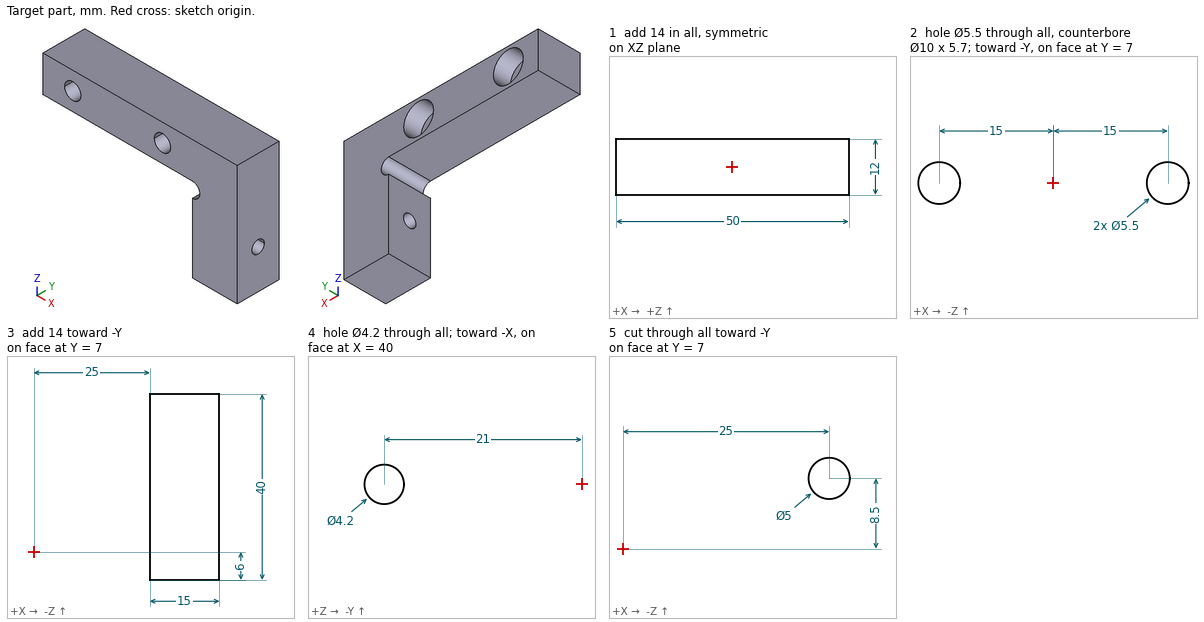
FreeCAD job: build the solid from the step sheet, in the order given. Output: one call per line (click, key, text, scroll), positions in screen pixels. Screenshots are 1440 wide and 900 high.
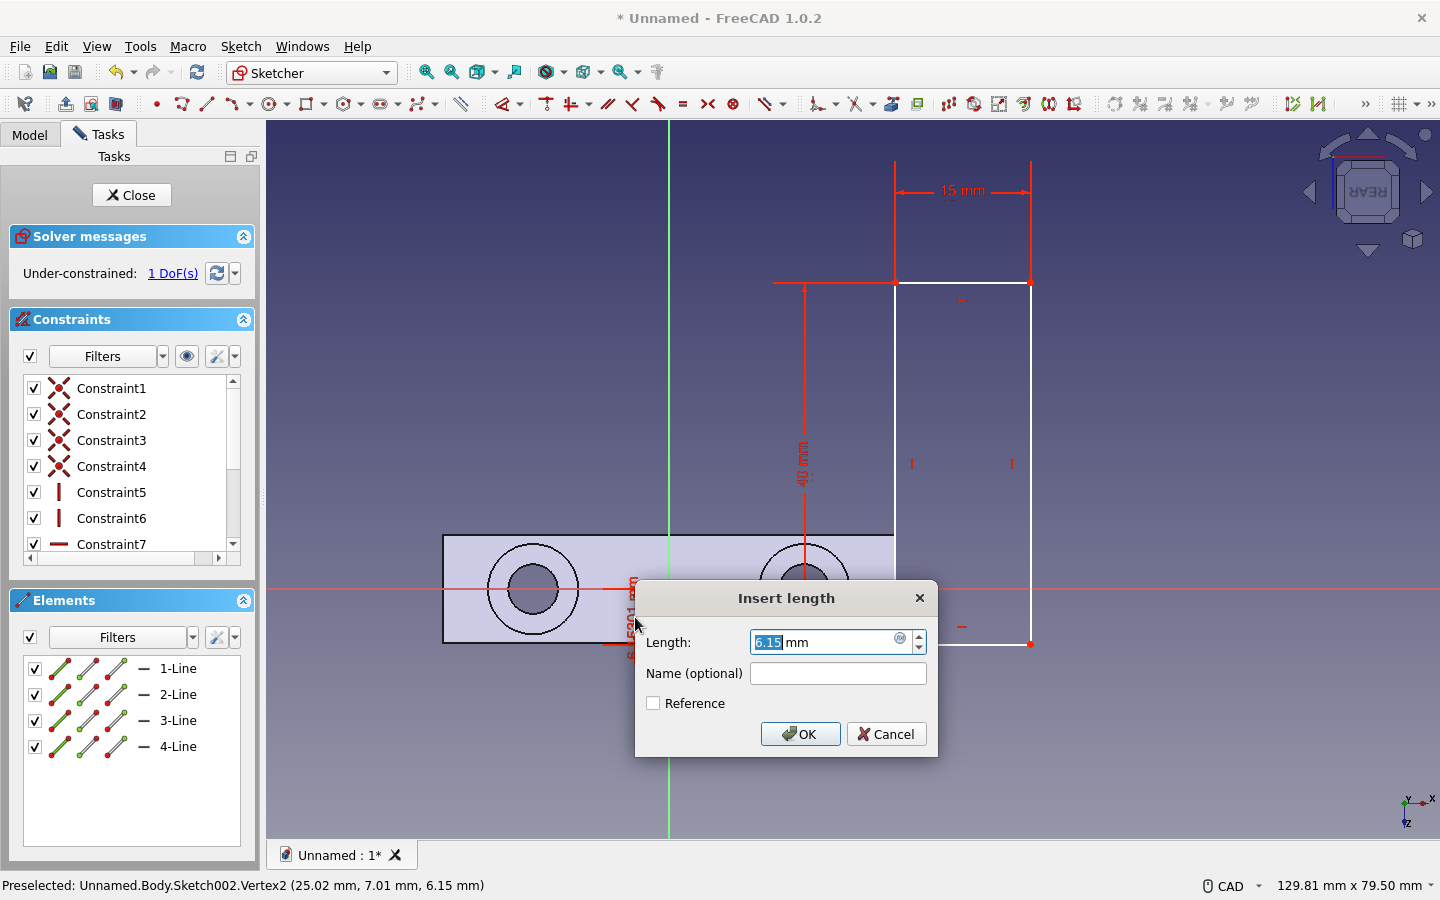
text(6)
key(Return)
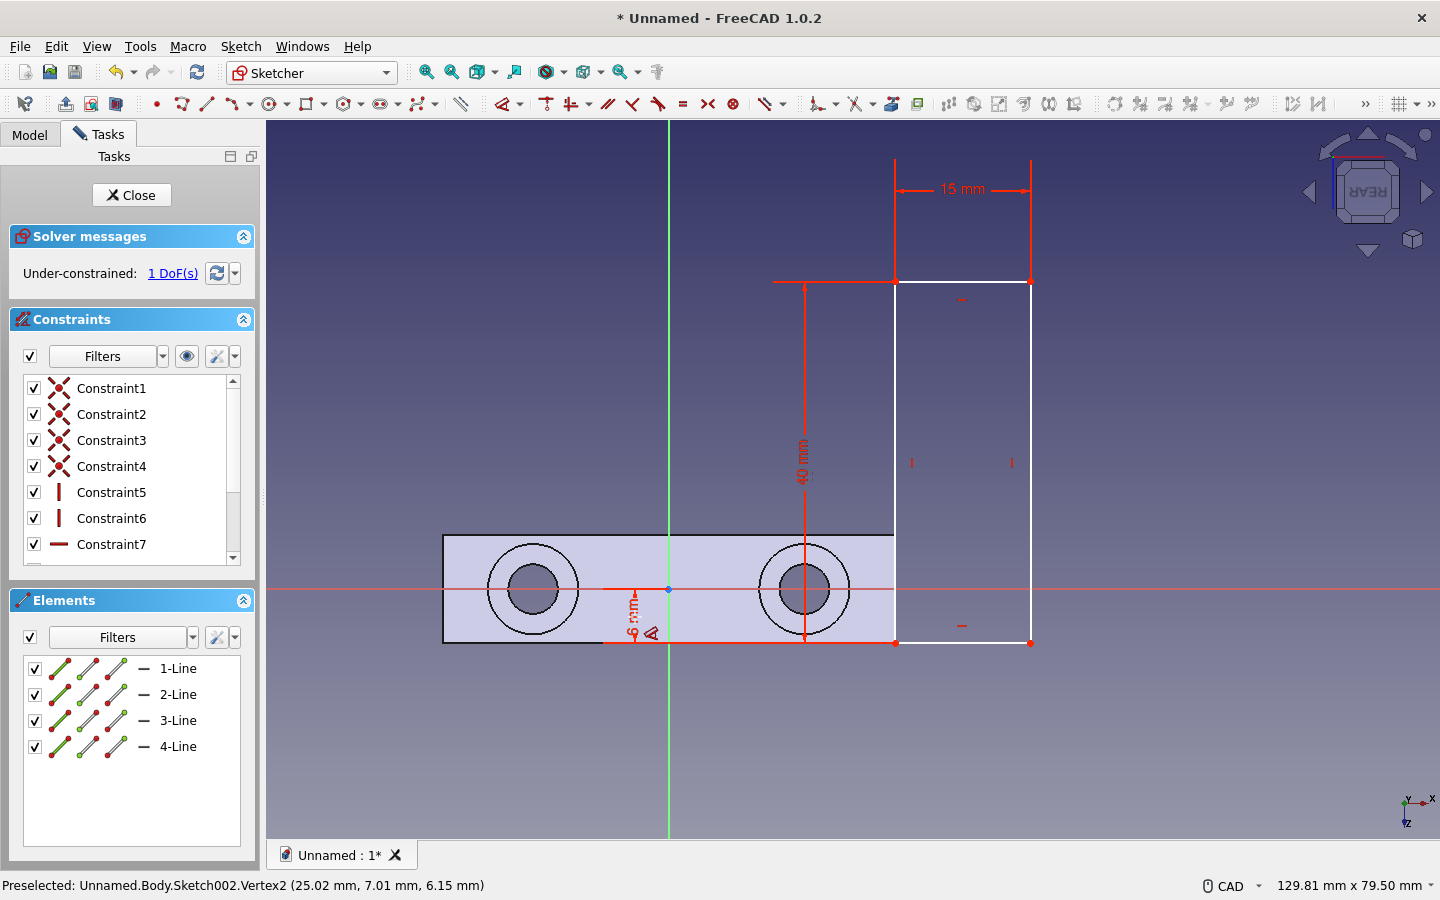
click(895, 282)
click(782, 248)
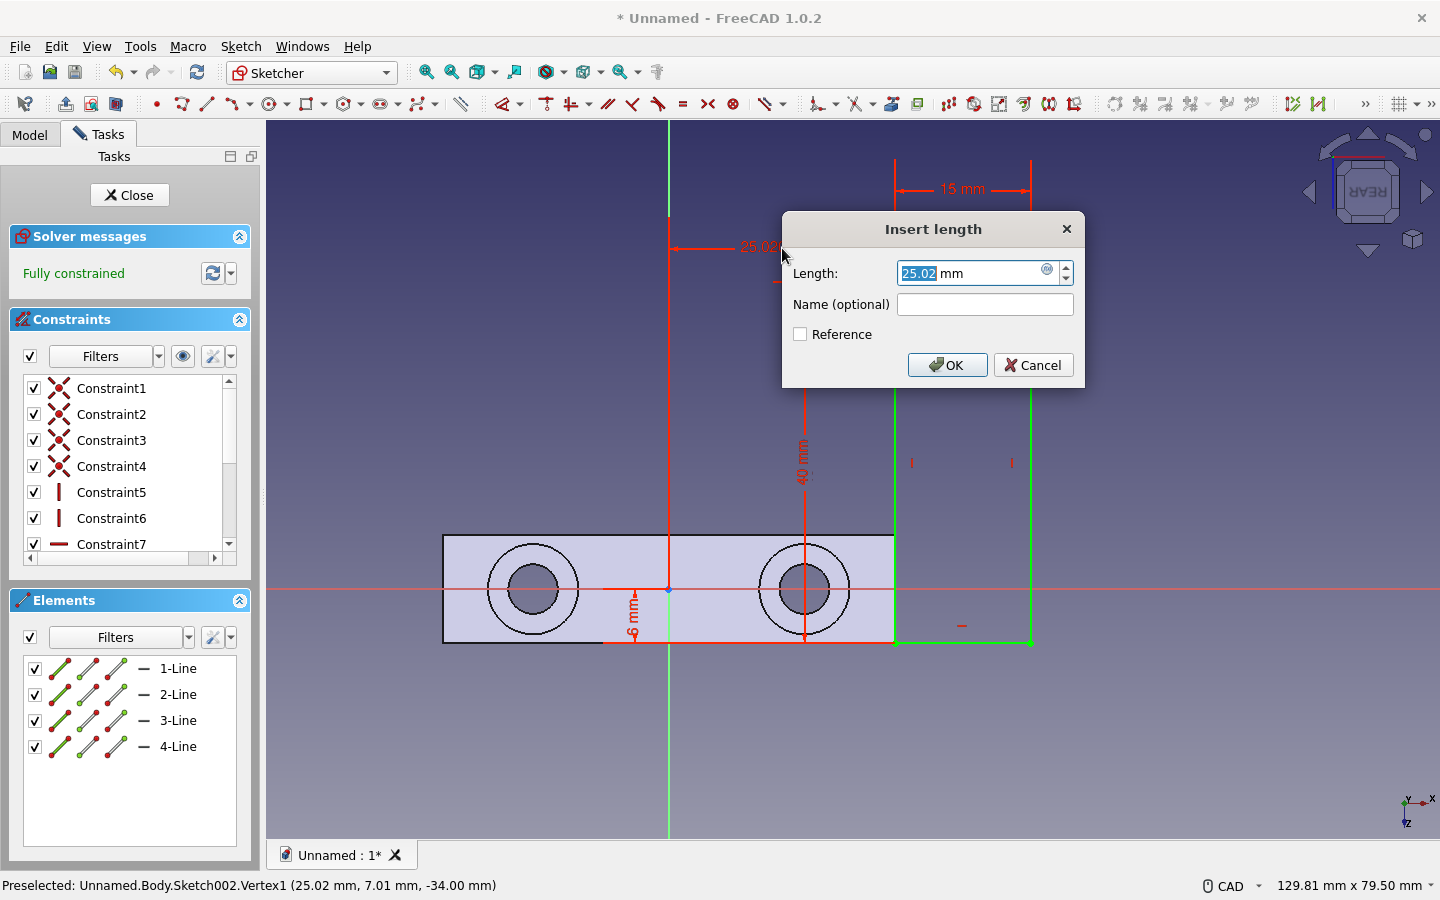
text(25)
key(Return)
key(Escape)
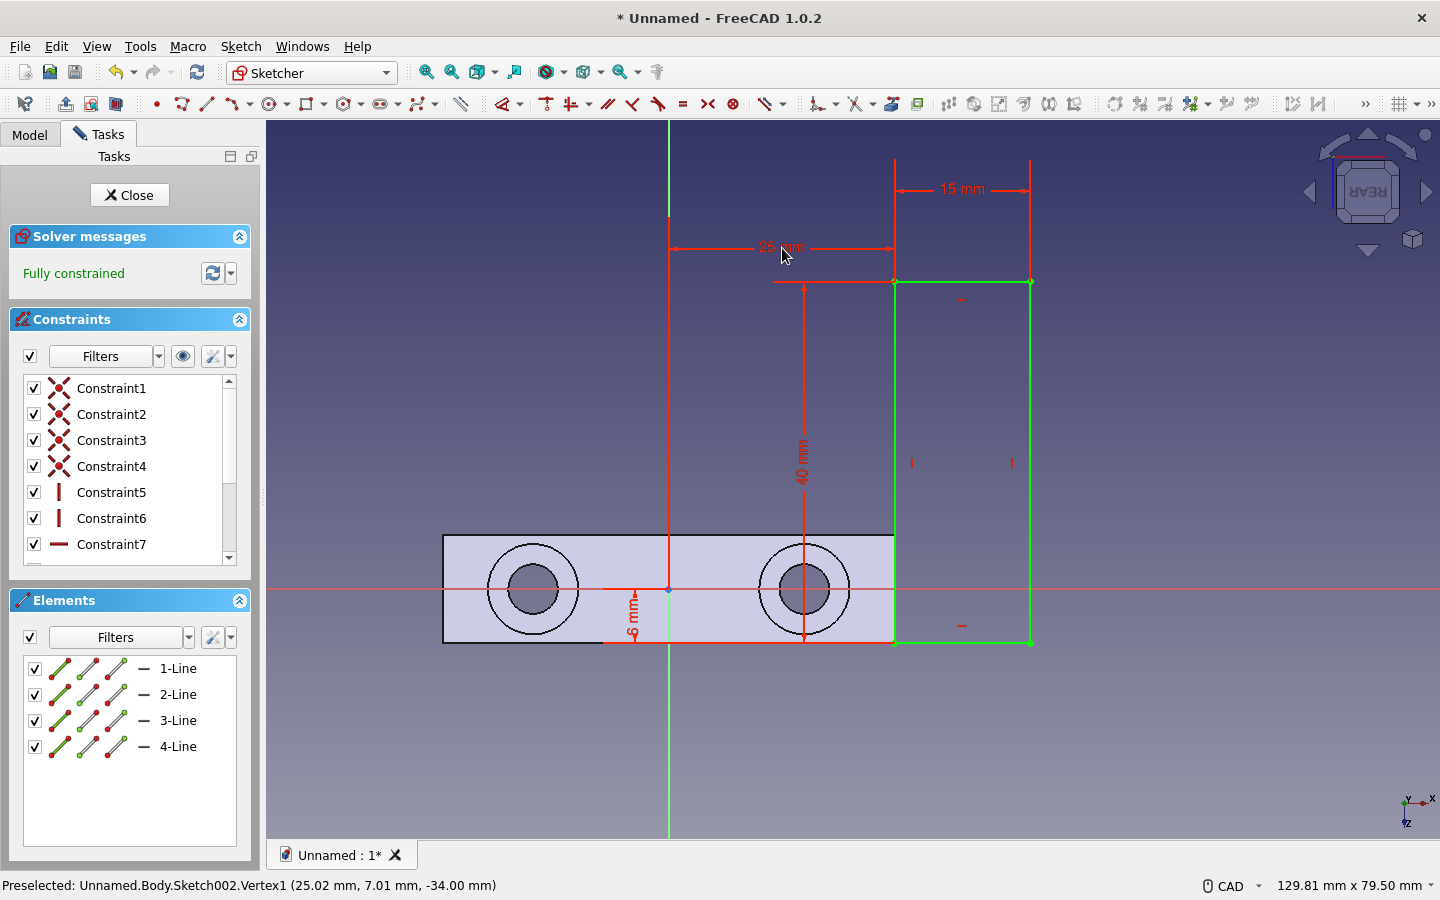
click(130, 195)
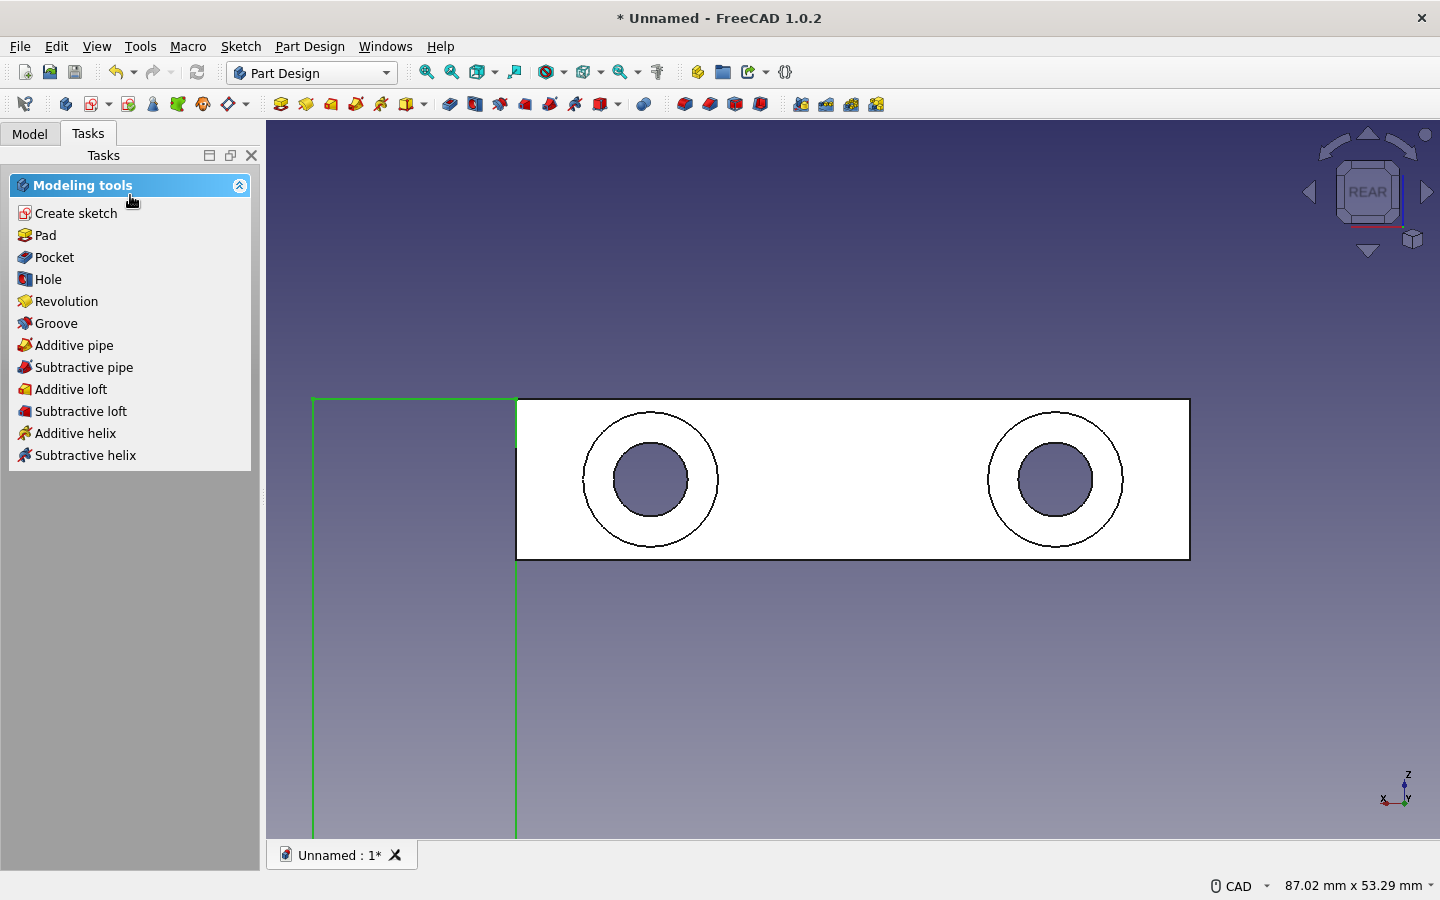
click(281, 104)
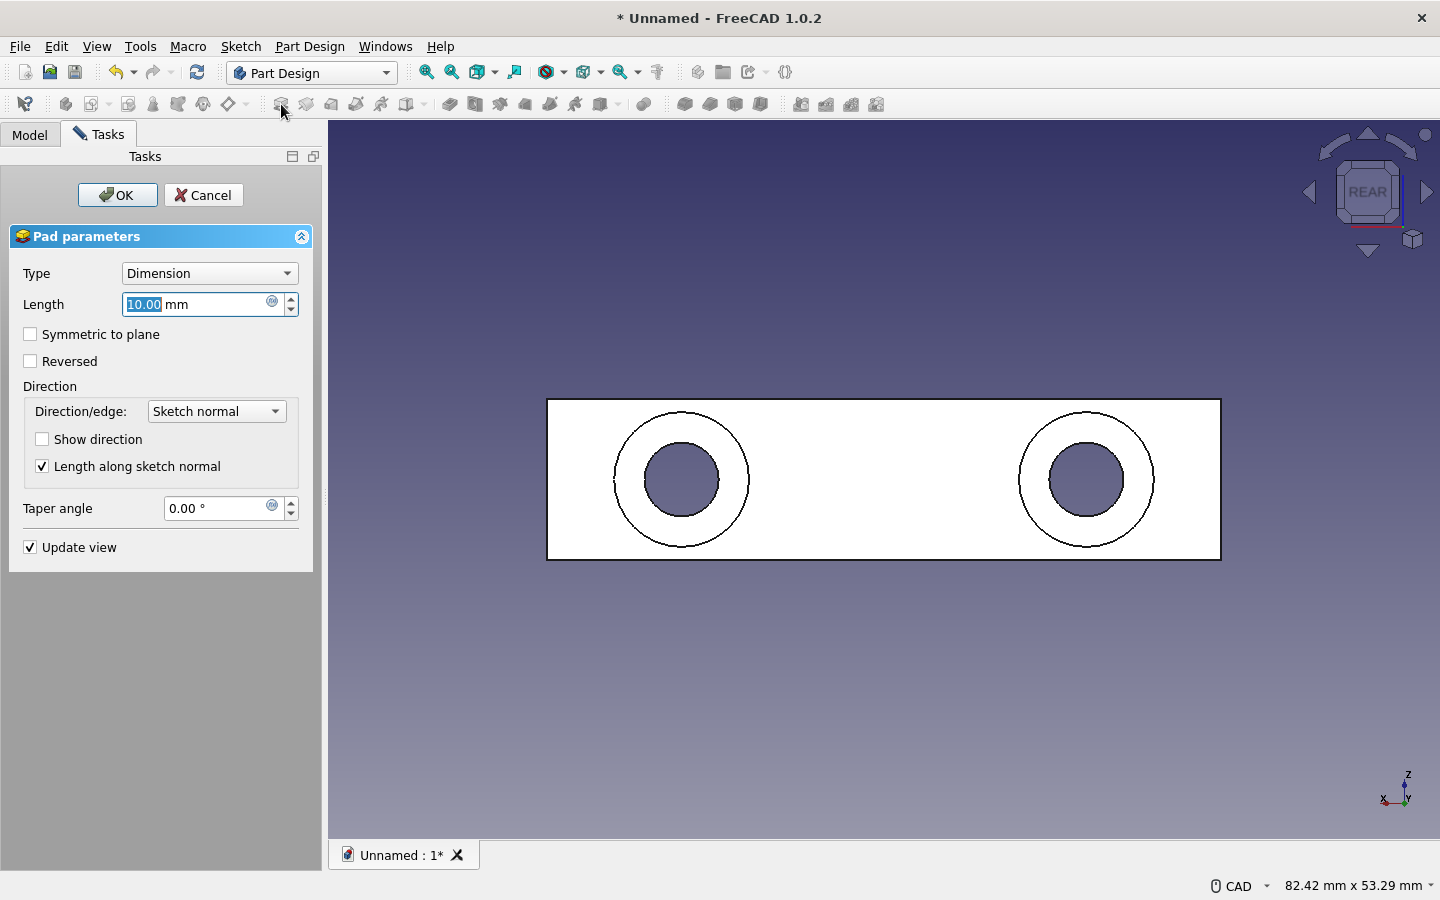
text(14)
key(Tab)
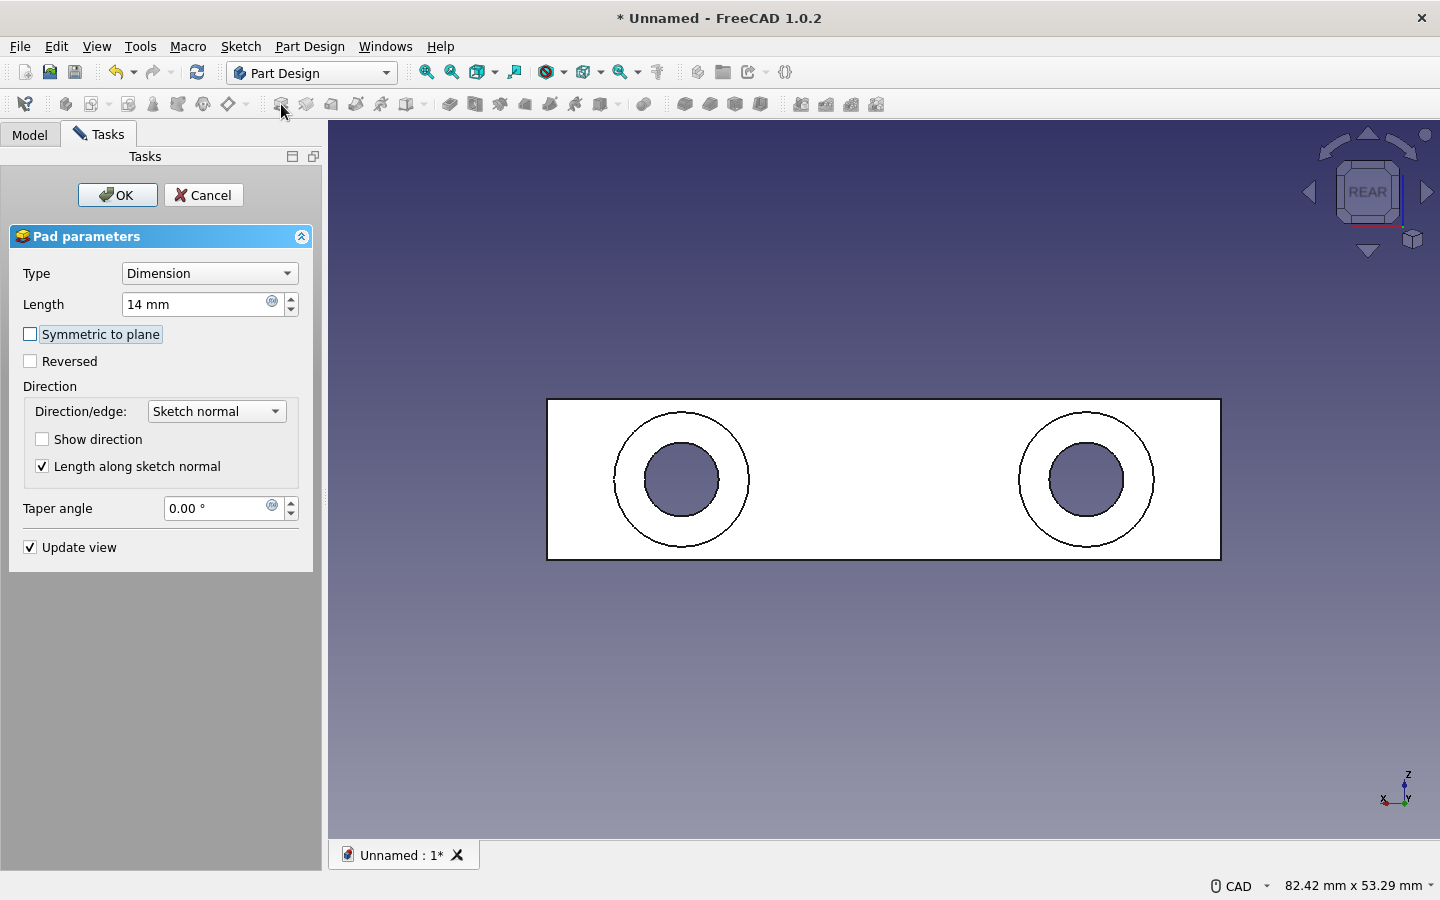
click(31, 361)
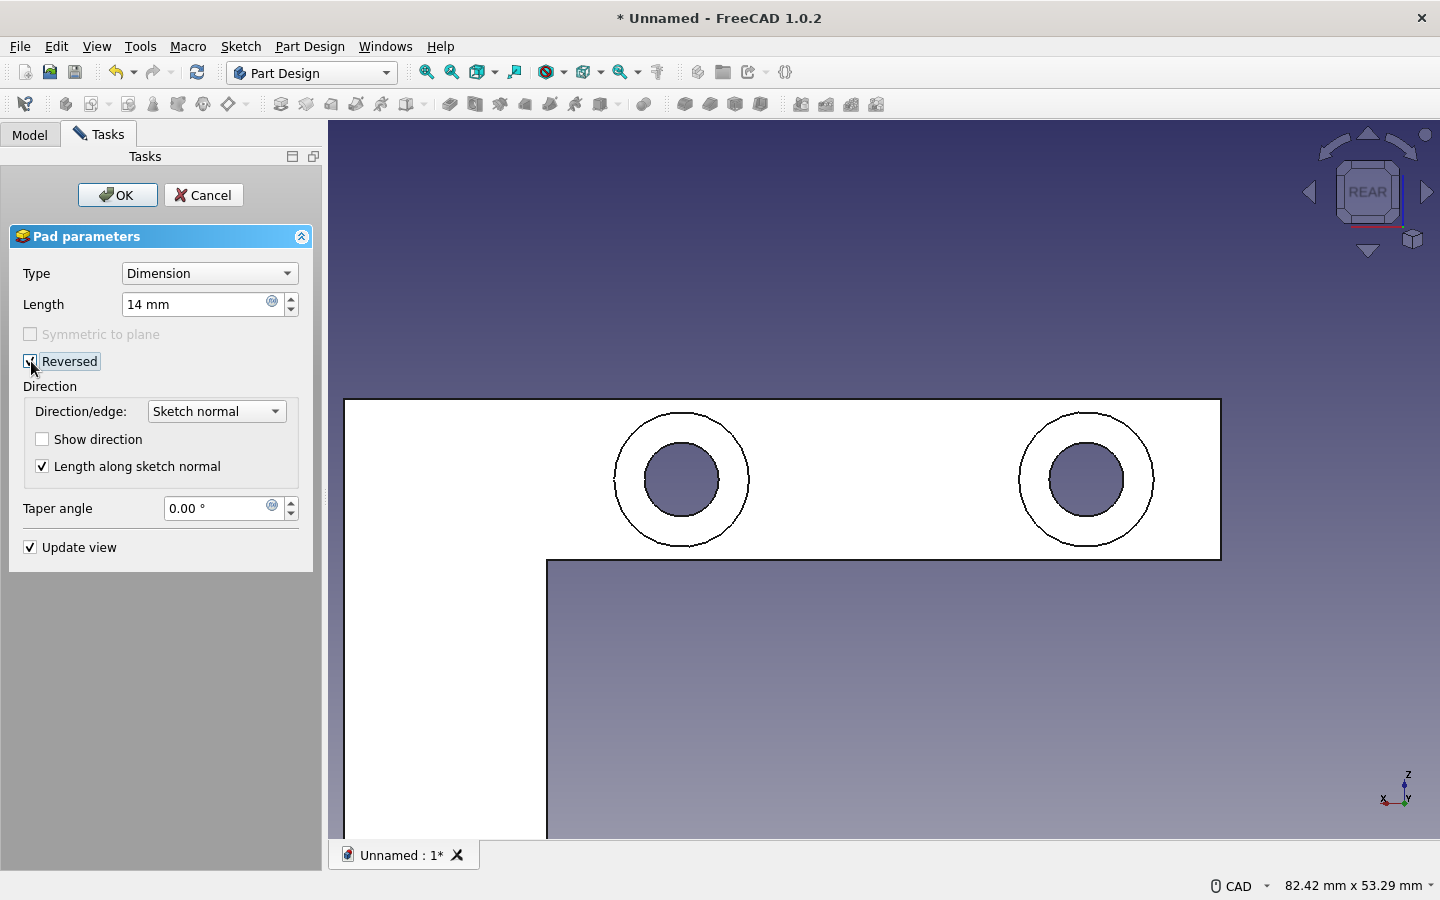
click(118, 195)